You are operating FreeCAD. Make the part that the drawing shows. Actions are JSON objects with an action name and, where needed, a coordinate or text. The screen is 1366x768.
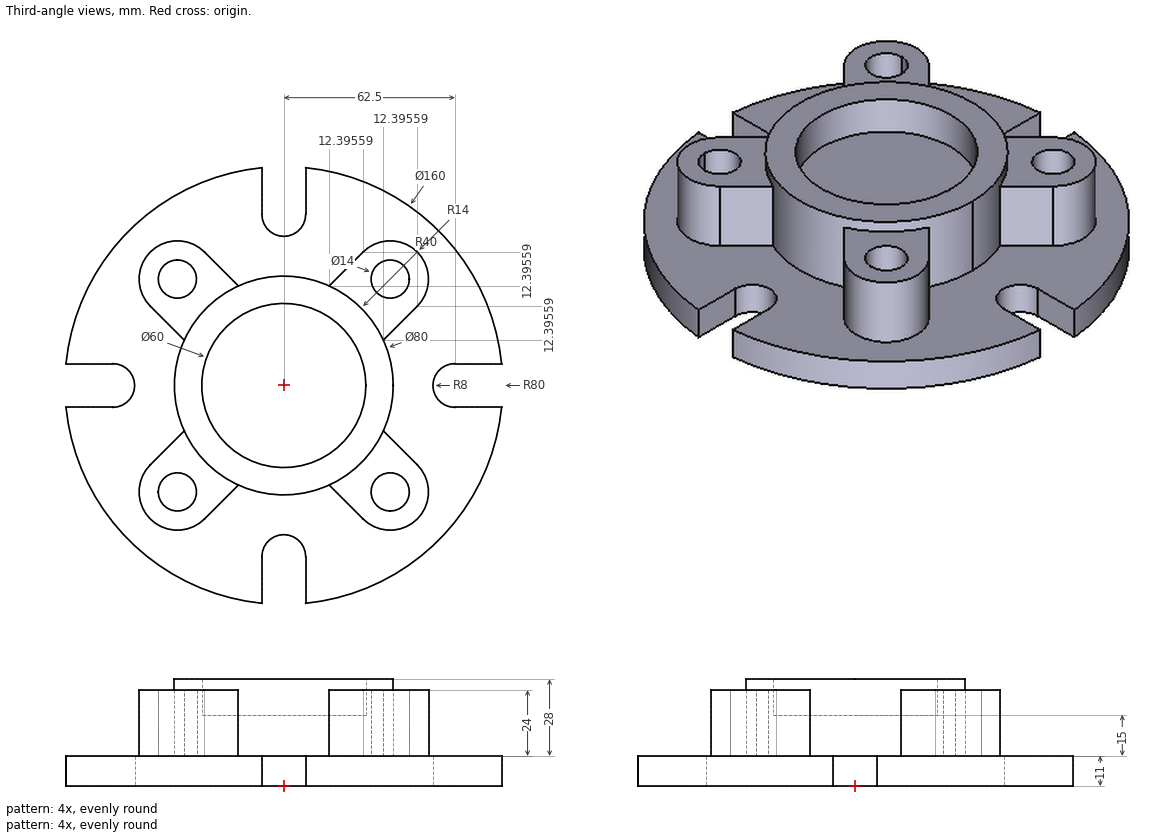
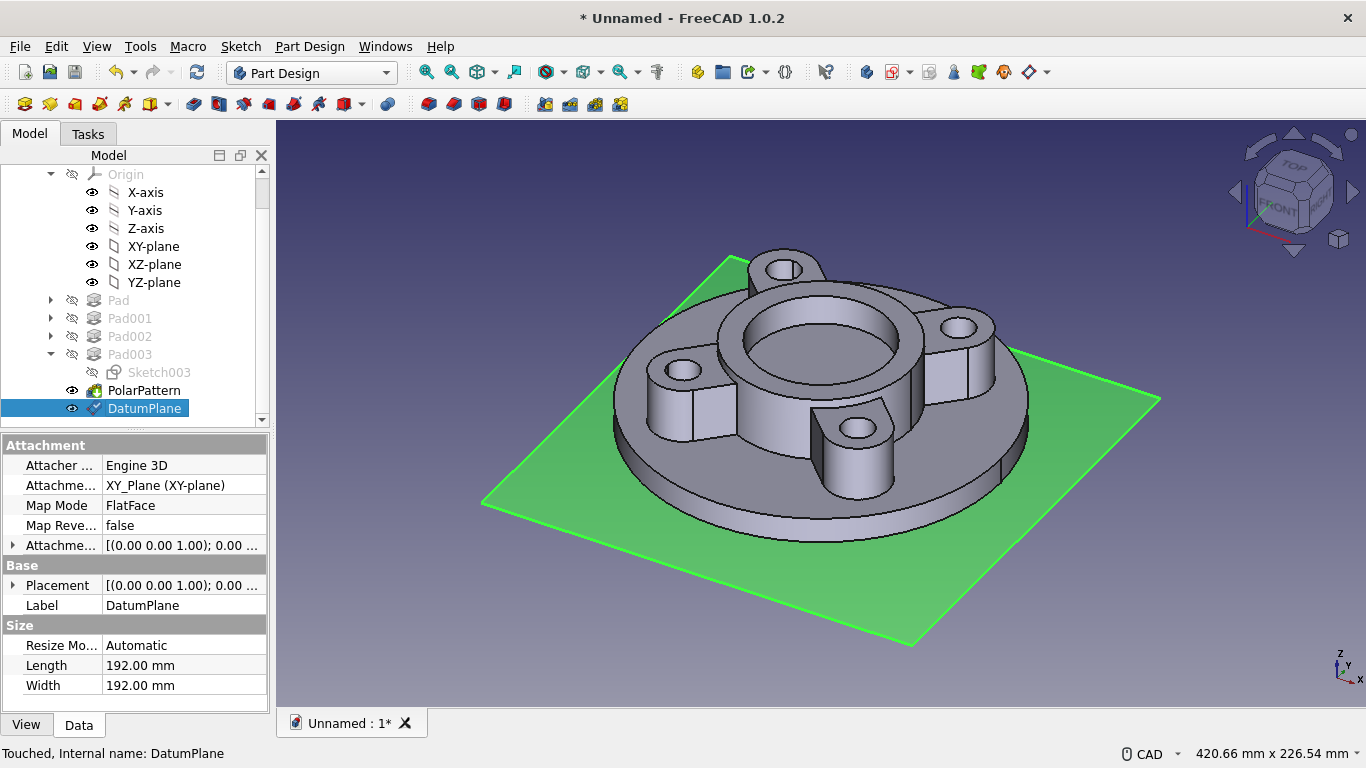
{"action": "left_click", "coordinate": [892, 72]}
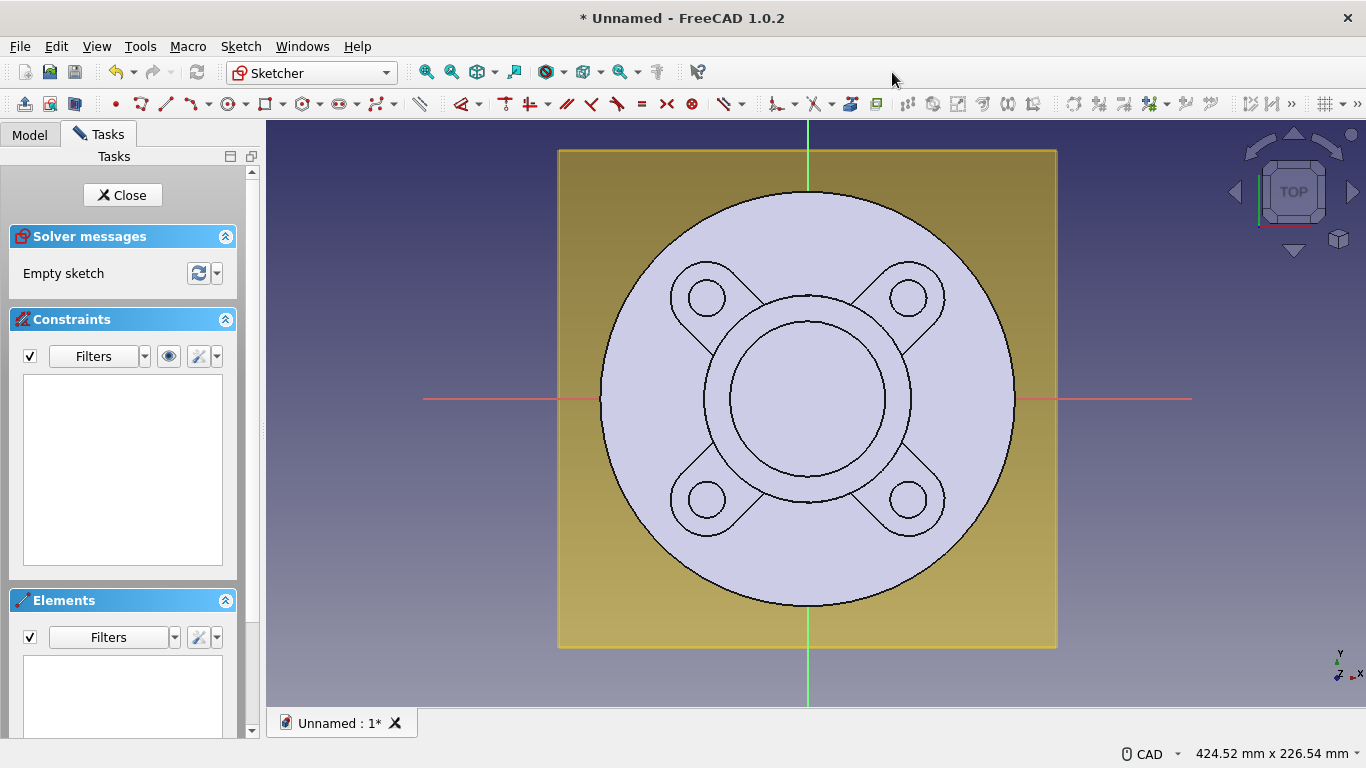
{"action": "key", "text": "q s"}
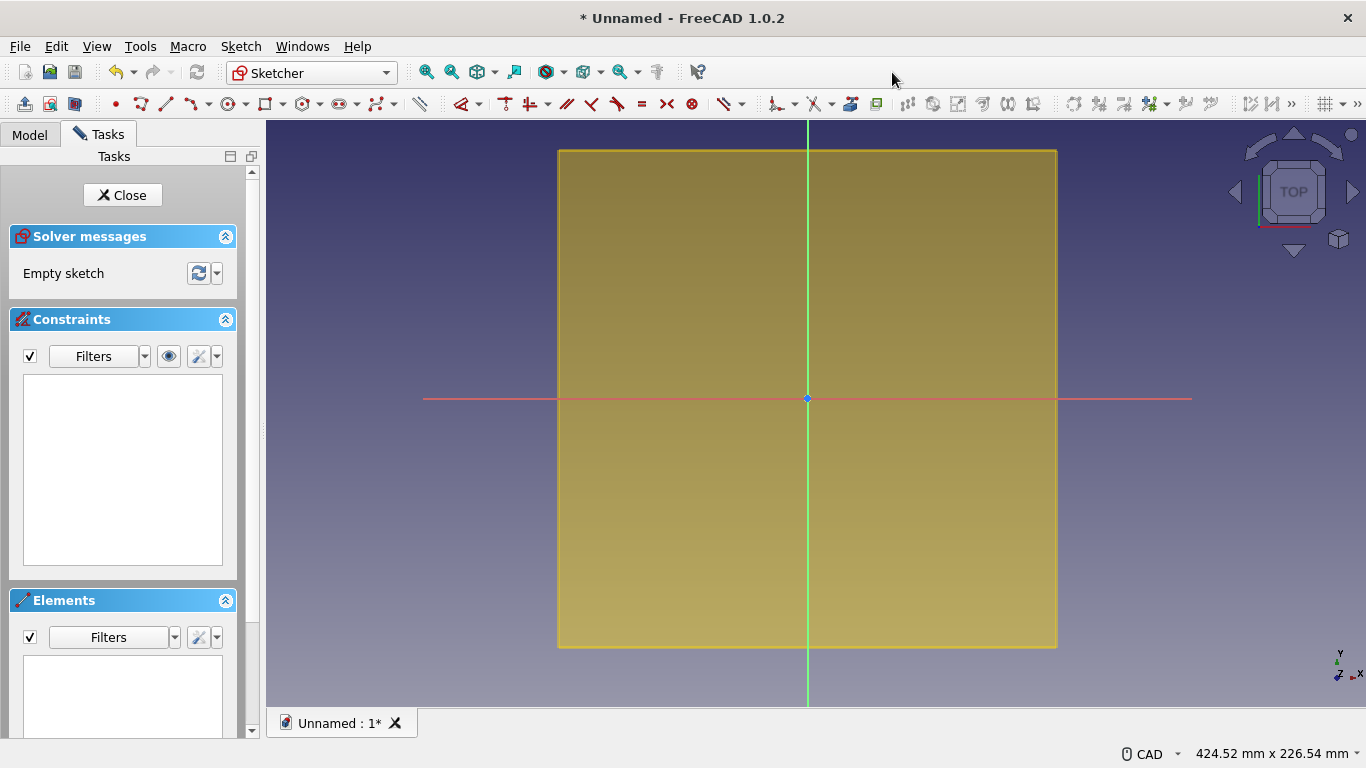
{"action": "scroll", "coordinate": [1011, 397], "scroll_direction": "up", "scroll_amount": 11}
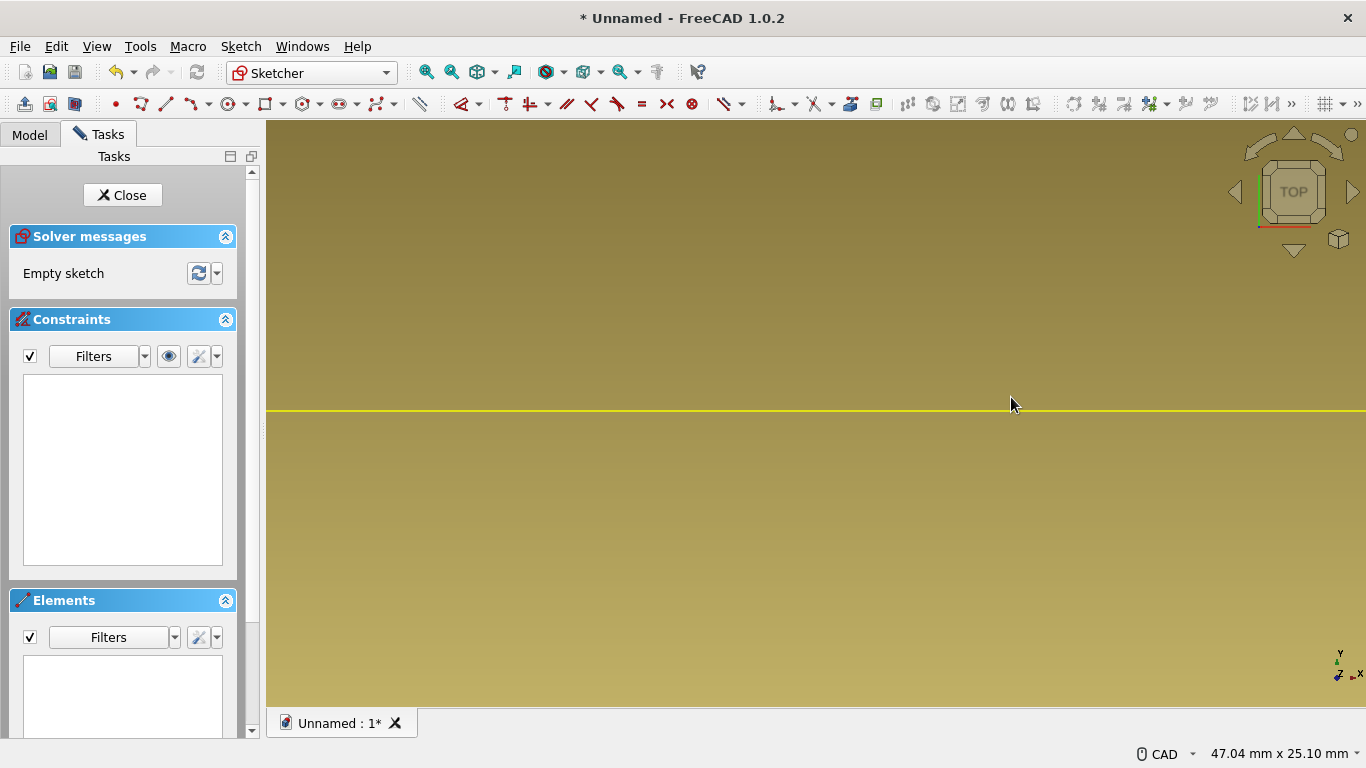
{"action": "key", "text": "g l"}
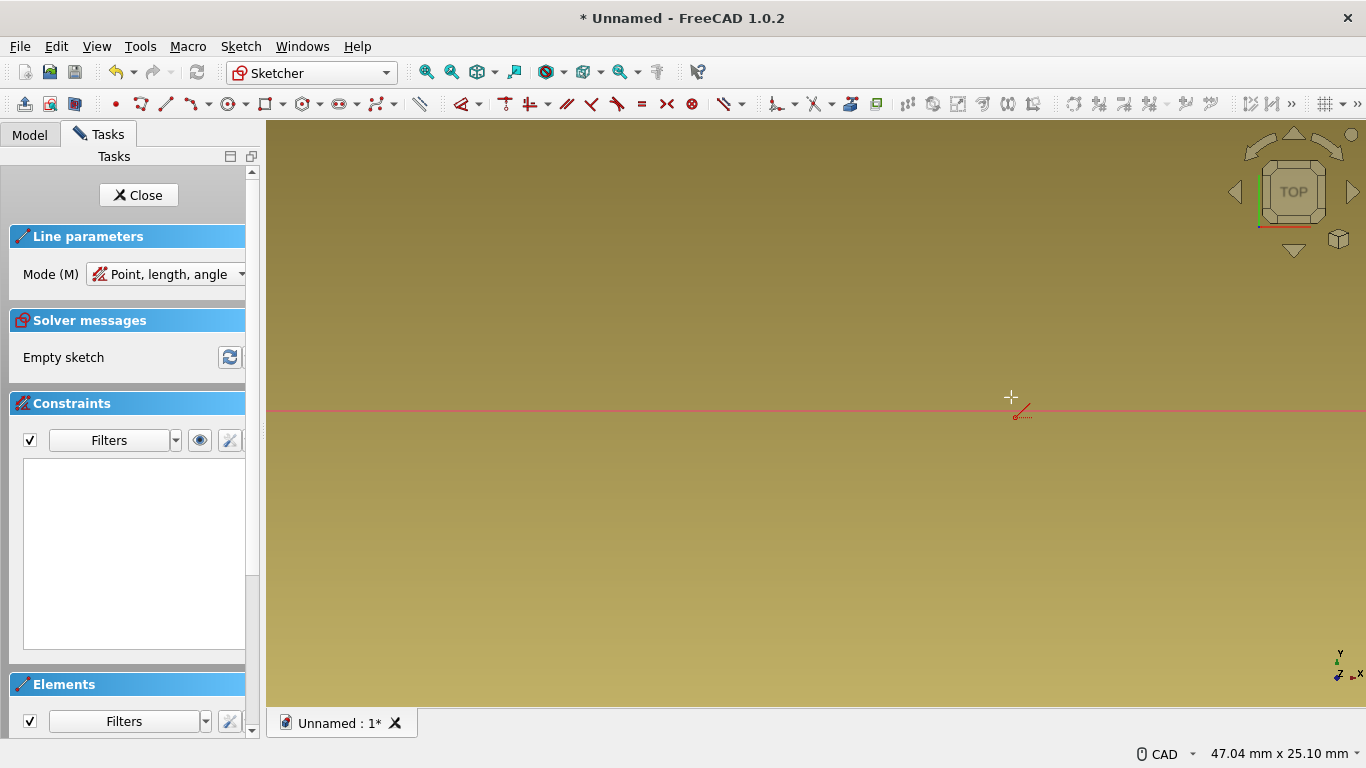
{"action": "left_click", "coordinate": [1032, 224]}
{"action": "left_click", "coordinate": [632, 224]}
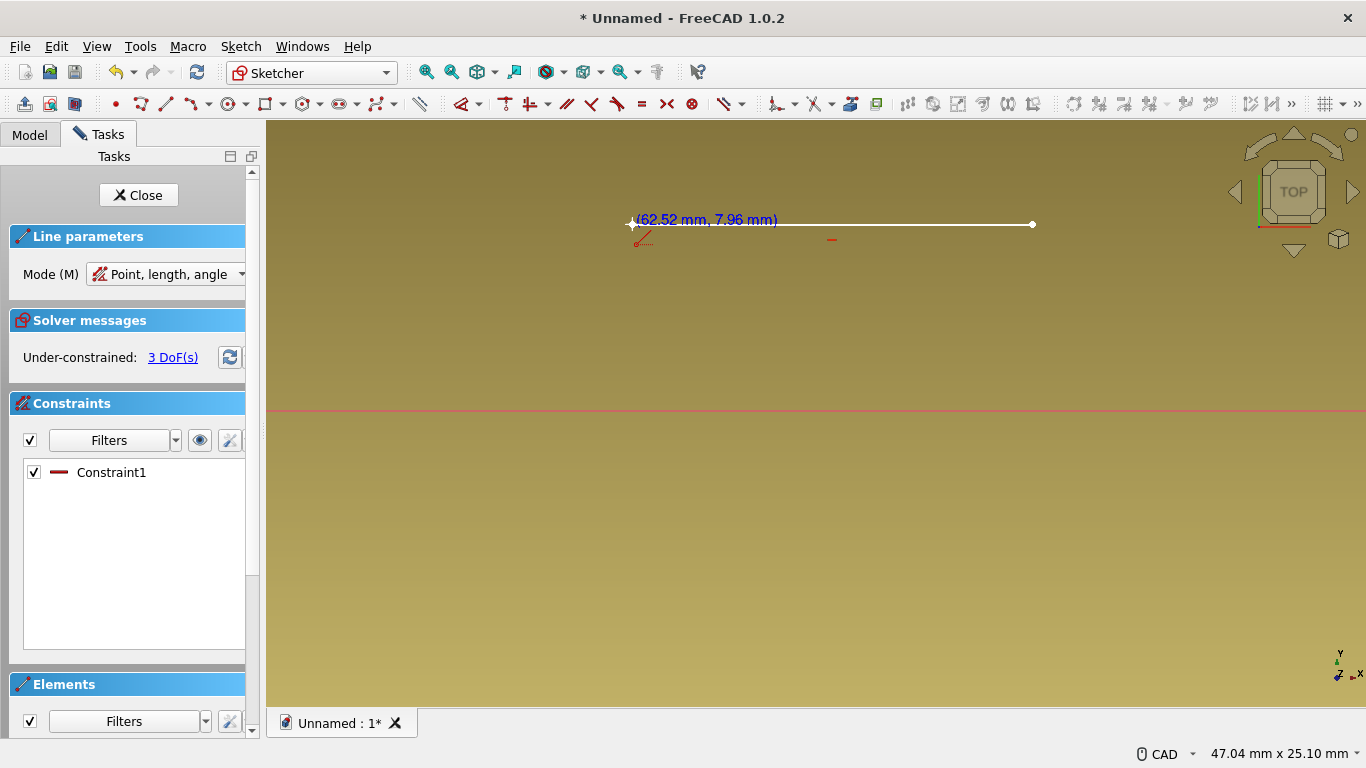
{"action": "left_click", "coordinate": [632, 598]}
{"action": "left_click", "coordinate": [1032, 598]}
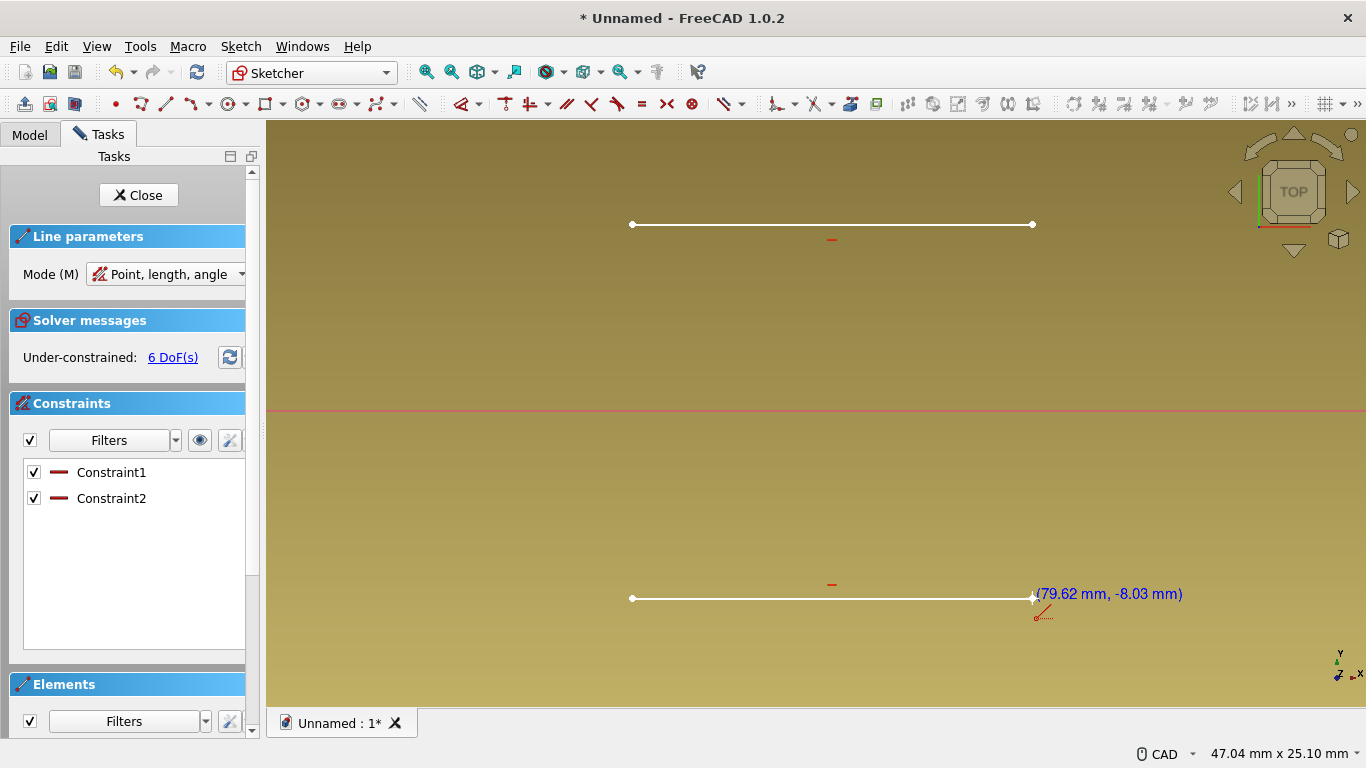
{"action": "left_click", "coordinate": [190, 104]}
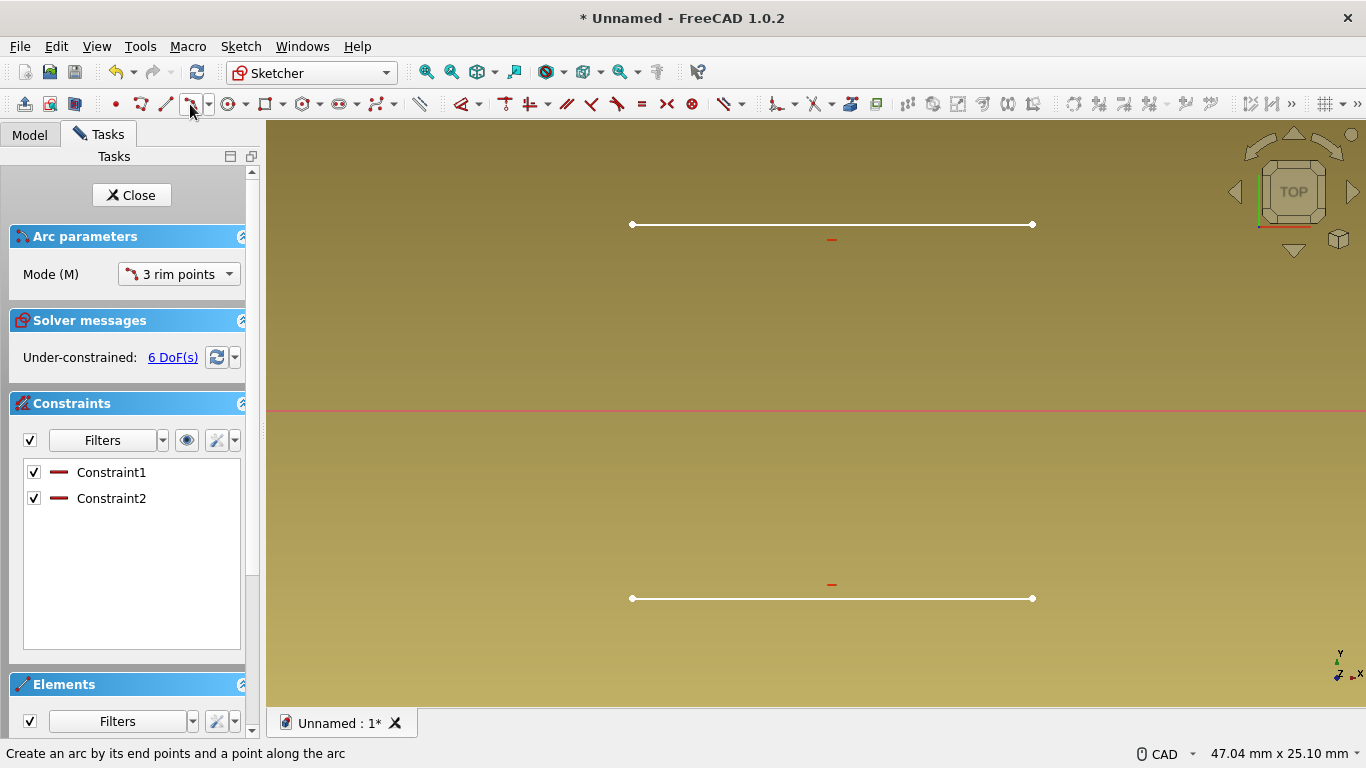
{"action": "left_click", "coordinate": [632, 225]}
{"action": "left_click", "coordinate": [632, 599]}
{"action": "left_click", "coordinate": [454, 353]}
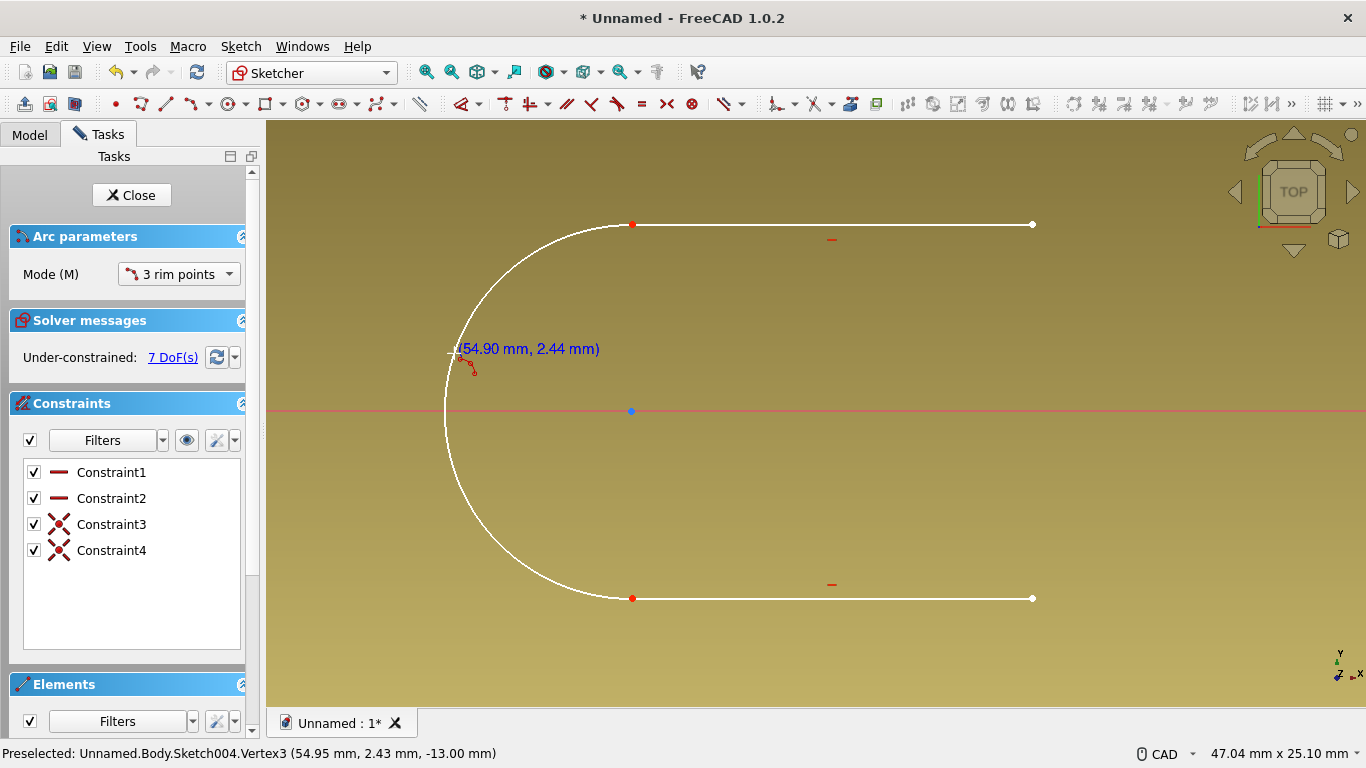
{"action": "left_click", "coordinate": [1032, 599]}
{"action": "left_click", "coordinate": [1032, 225]}